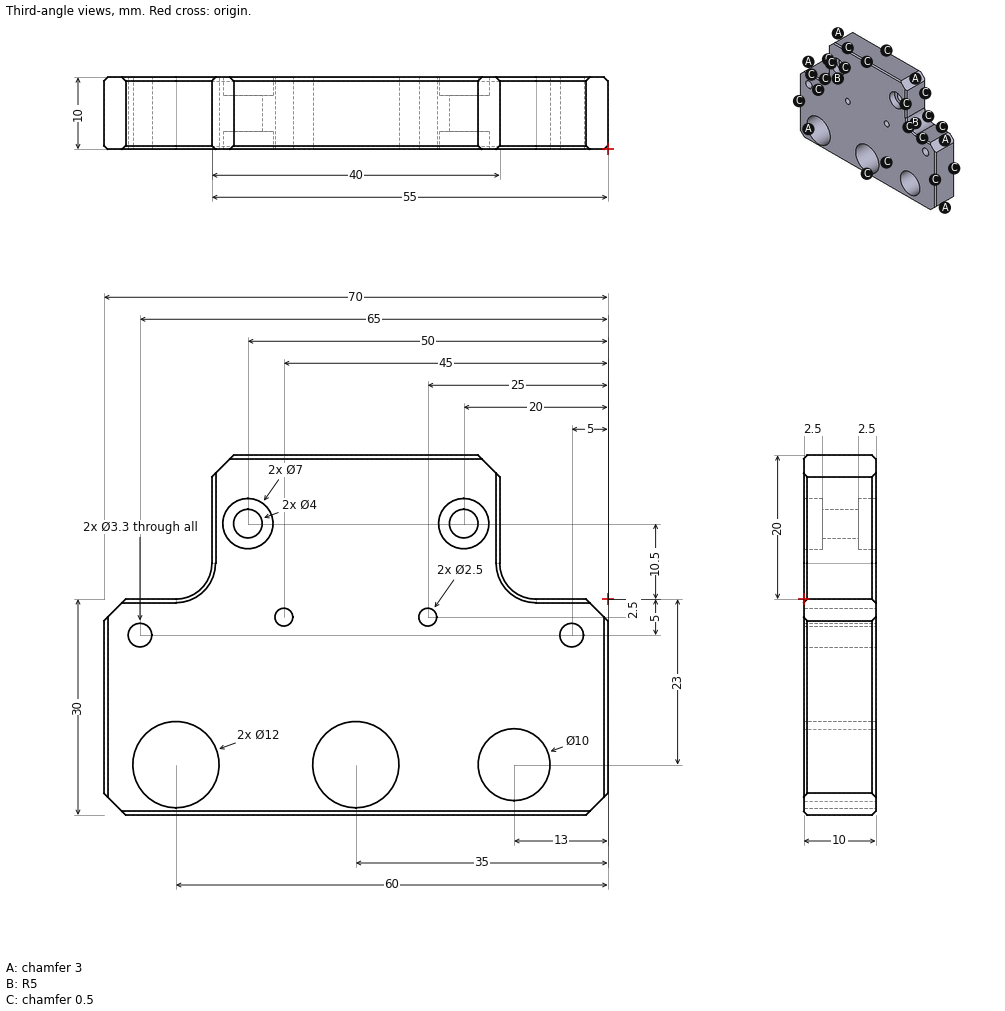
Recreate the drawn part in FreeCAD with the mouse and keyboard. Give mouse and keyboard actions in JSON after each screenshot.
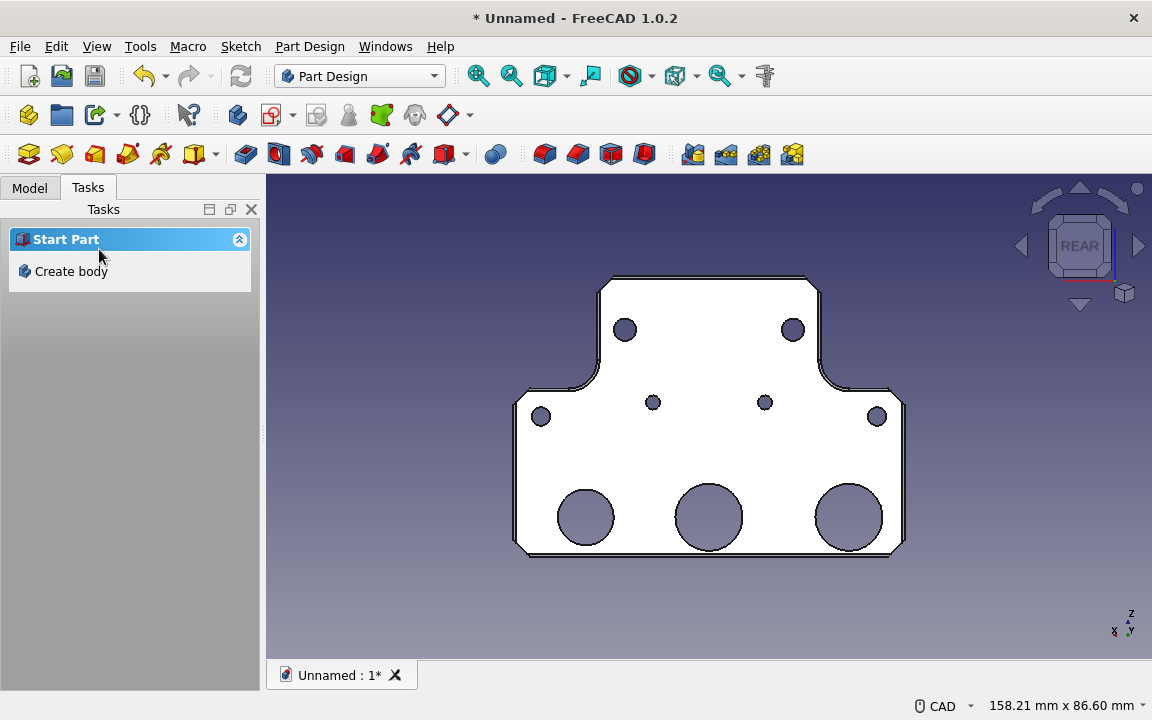
{"action": "left_click", "coordinate": [709, 337]}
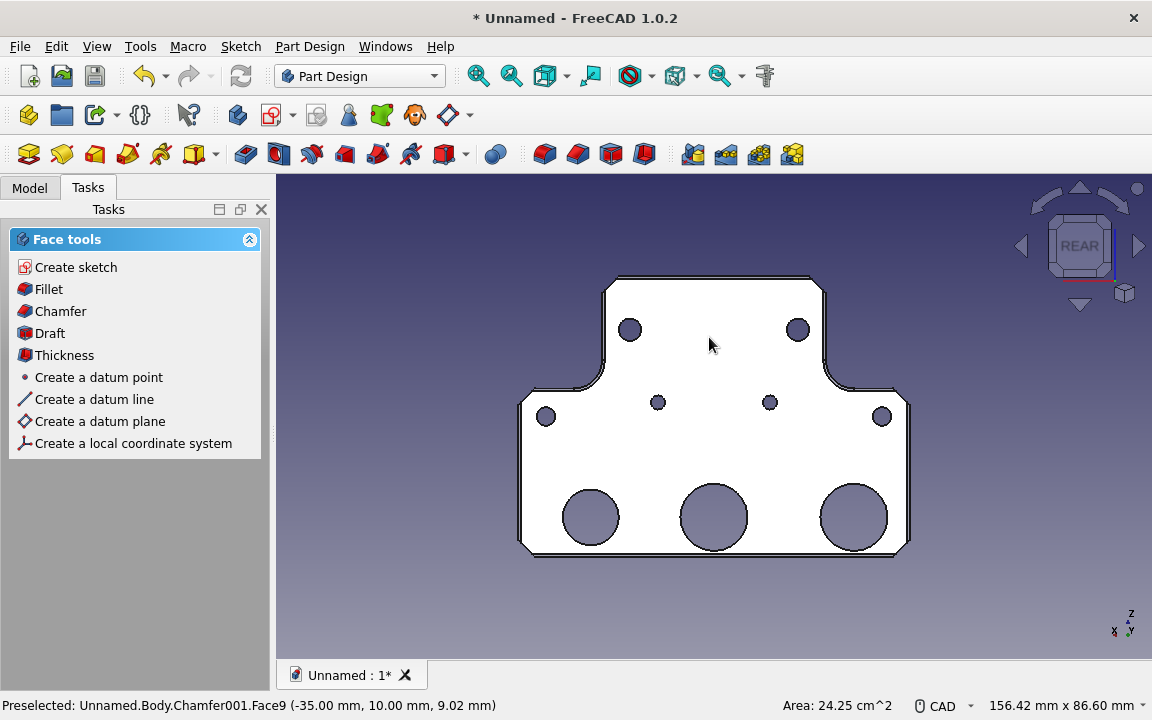
{"action": "left_click", "coordinate": [270, 116]}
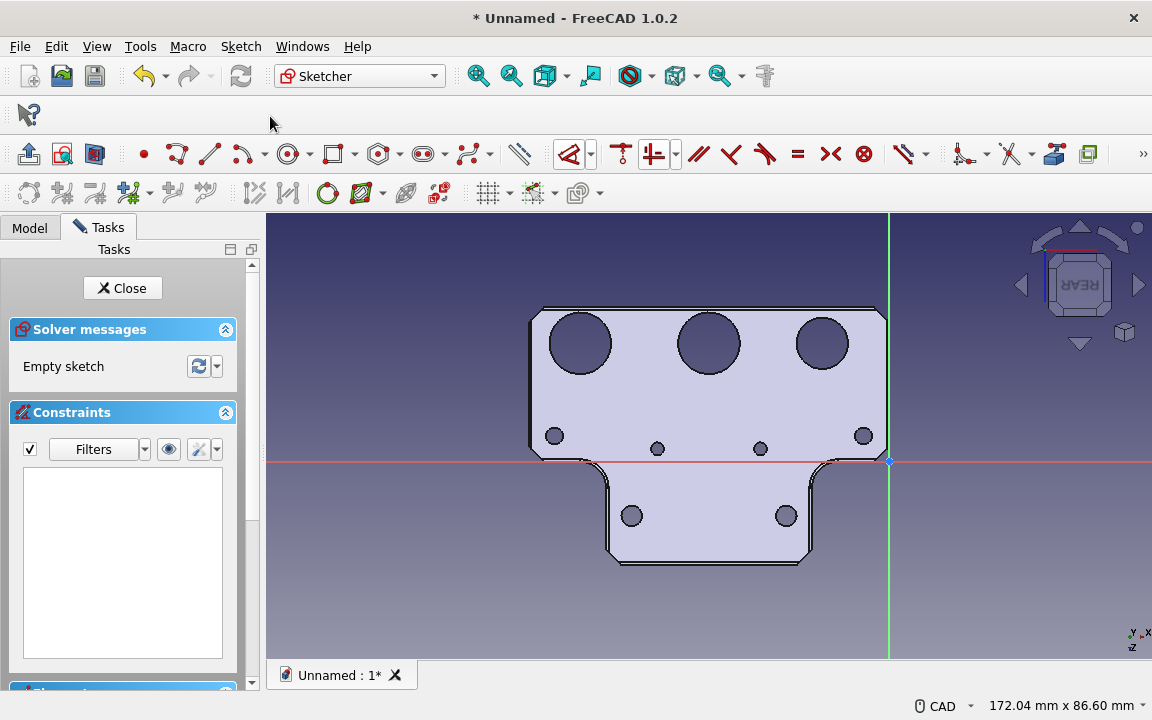
{"action": "scroll", "coordinate": [886, 573], "scroll_direction": "up", "scroll_amount": 3}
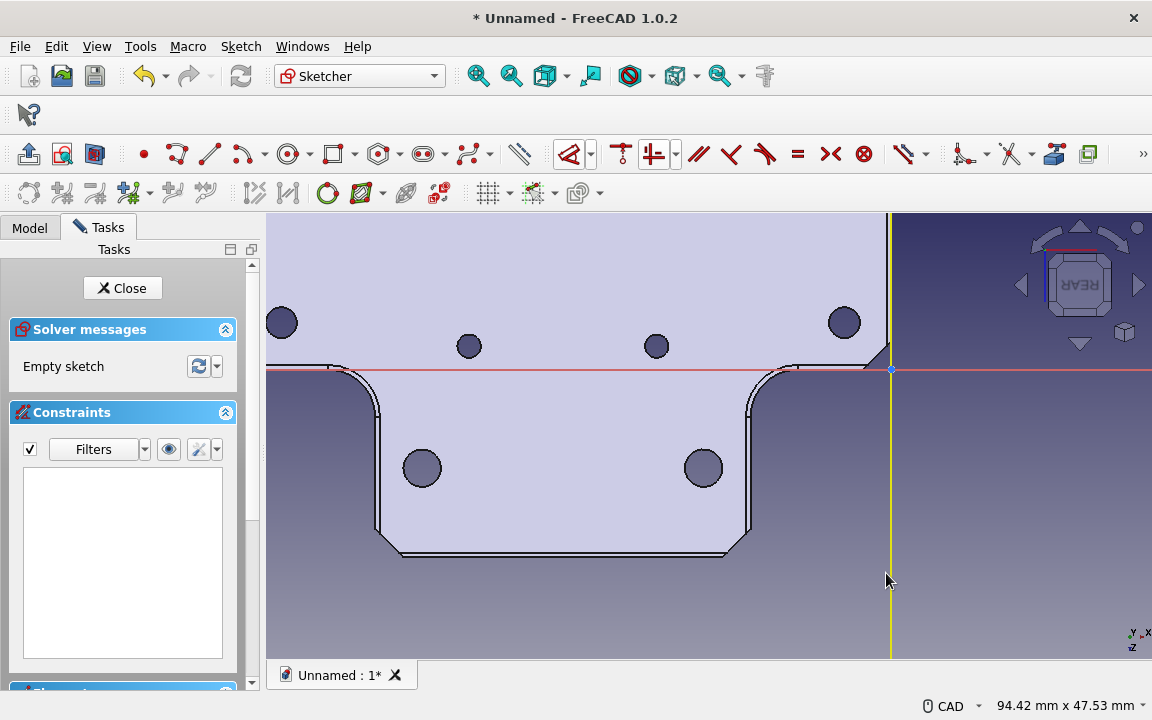
{"action": "left_click", "coordinate": [288, 154]}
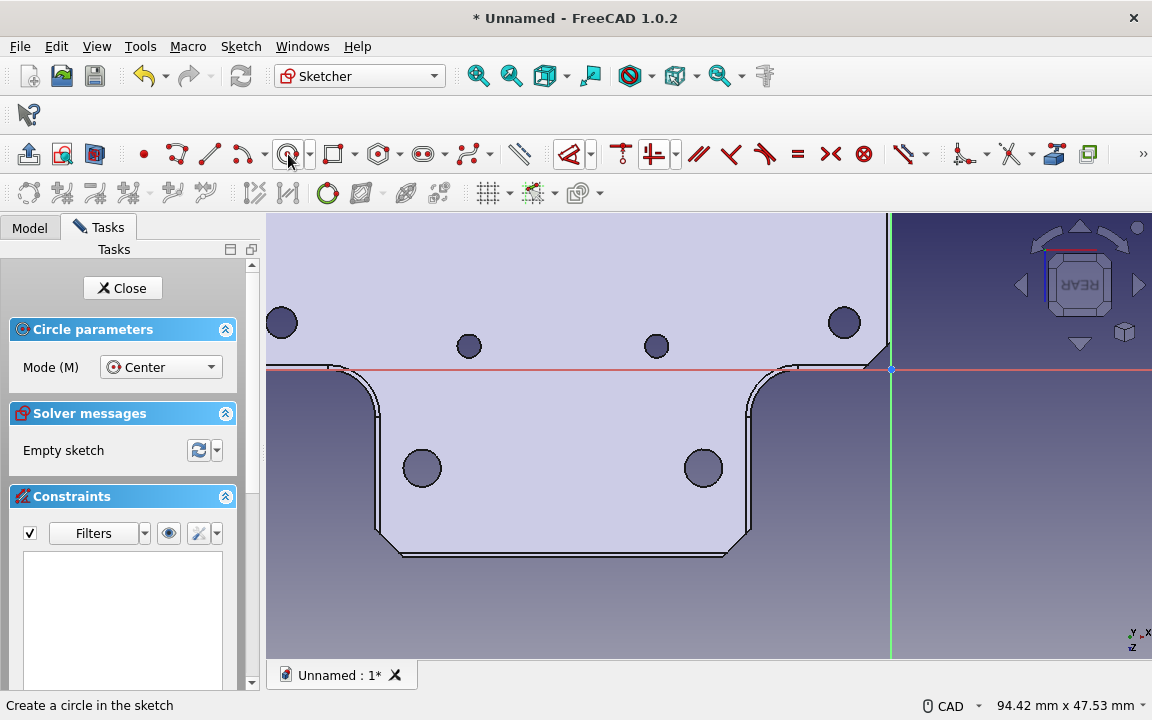
{"action": "left_click", "coordinate": [422, 468]}
{"action": "left_click", "coordinate": [445, 445]}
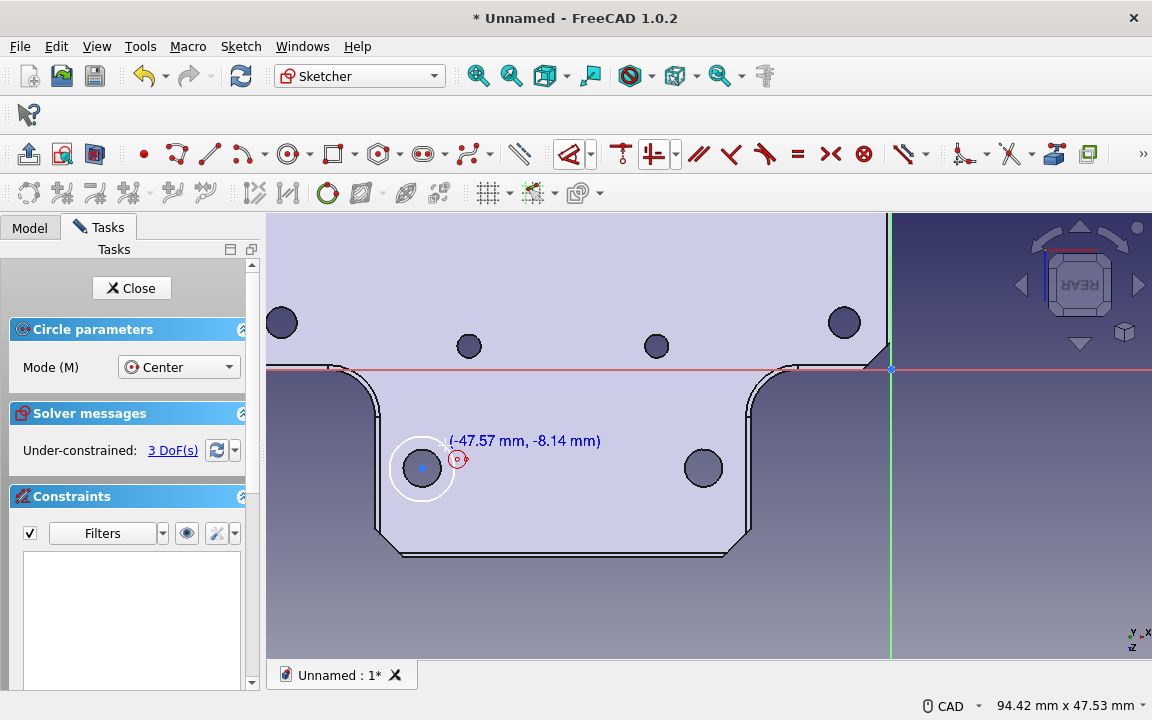
{"action": "left_click", "coordinate": [704, 468]}
{"action": "left_click", "coordinate": [727, 445]}
{"action": "key", "text": "Escape"}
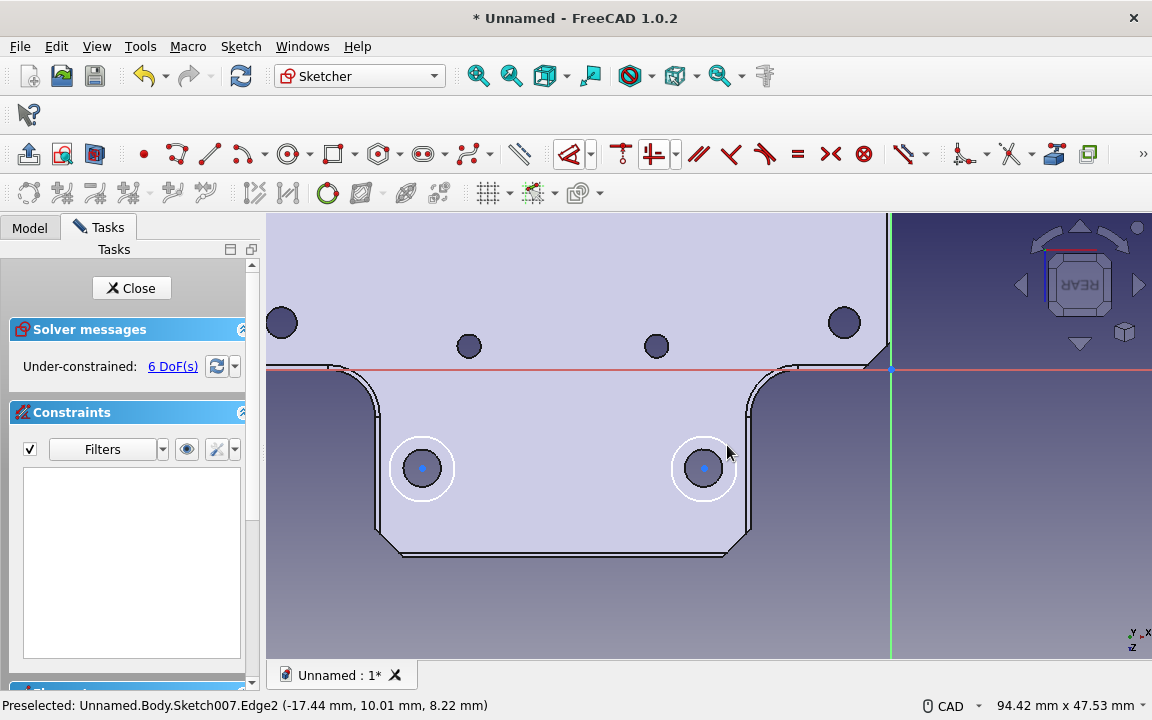
{"action": "left_click", "coordinate": [445, 446]}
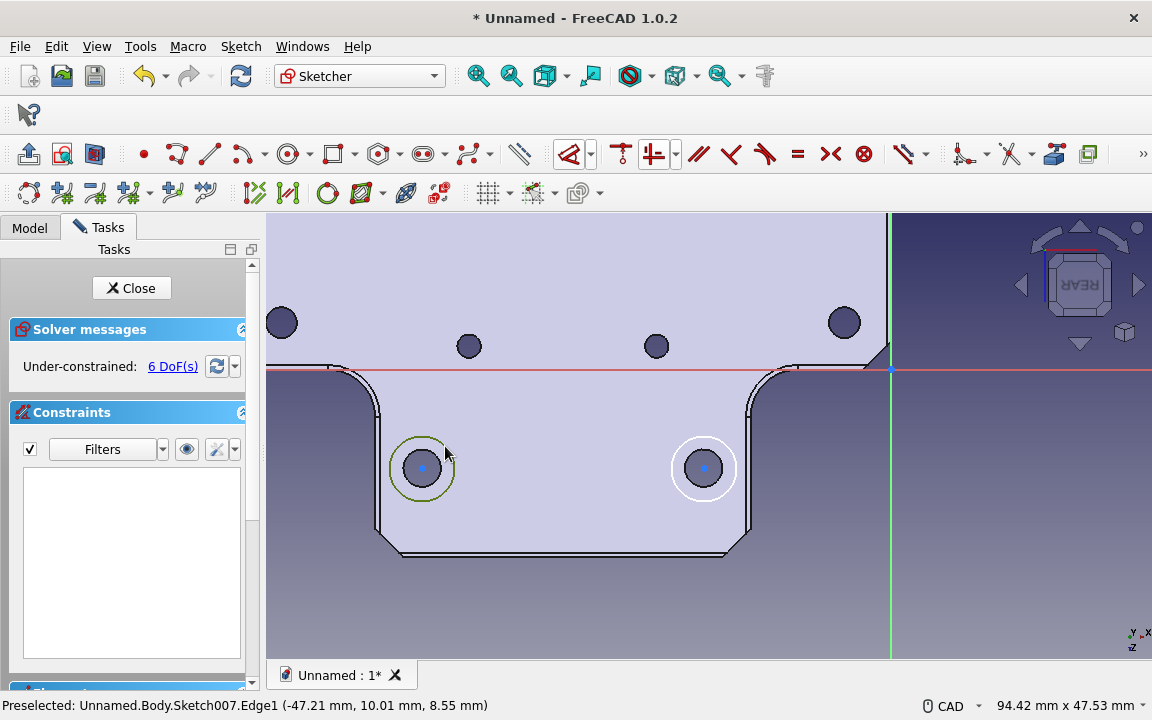
{"action": "left_click", "coordinate": [727, 446]}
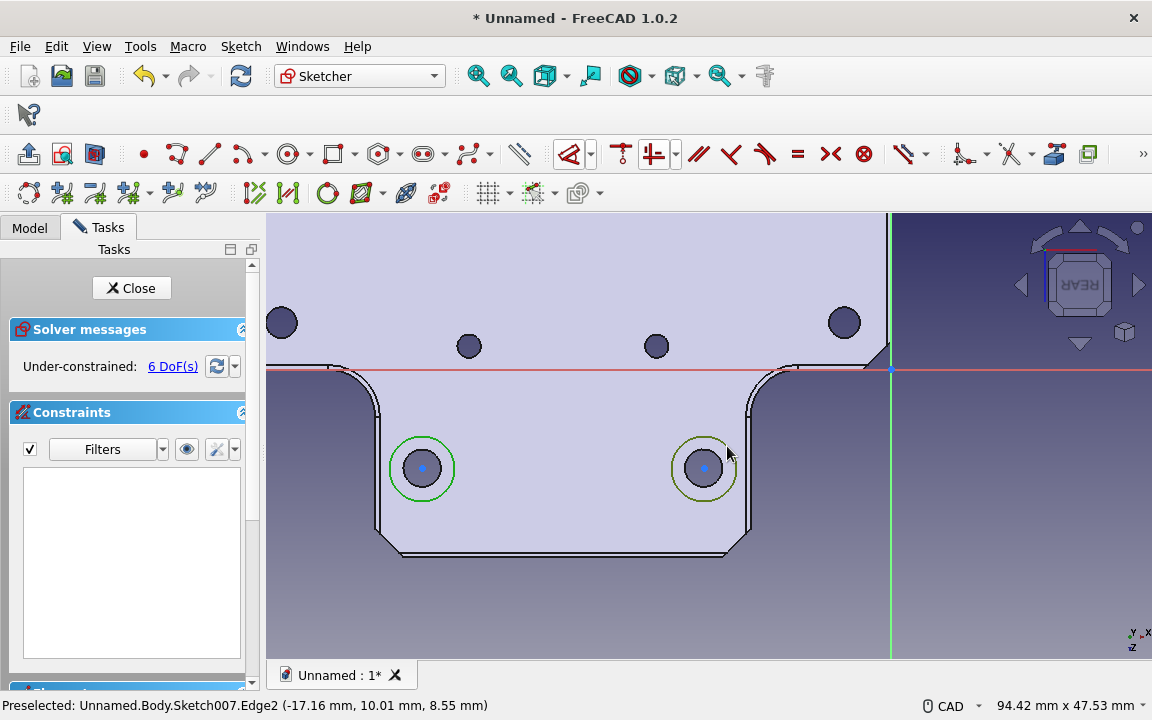
{"action": "left_click", "coordinate": [798, 154]}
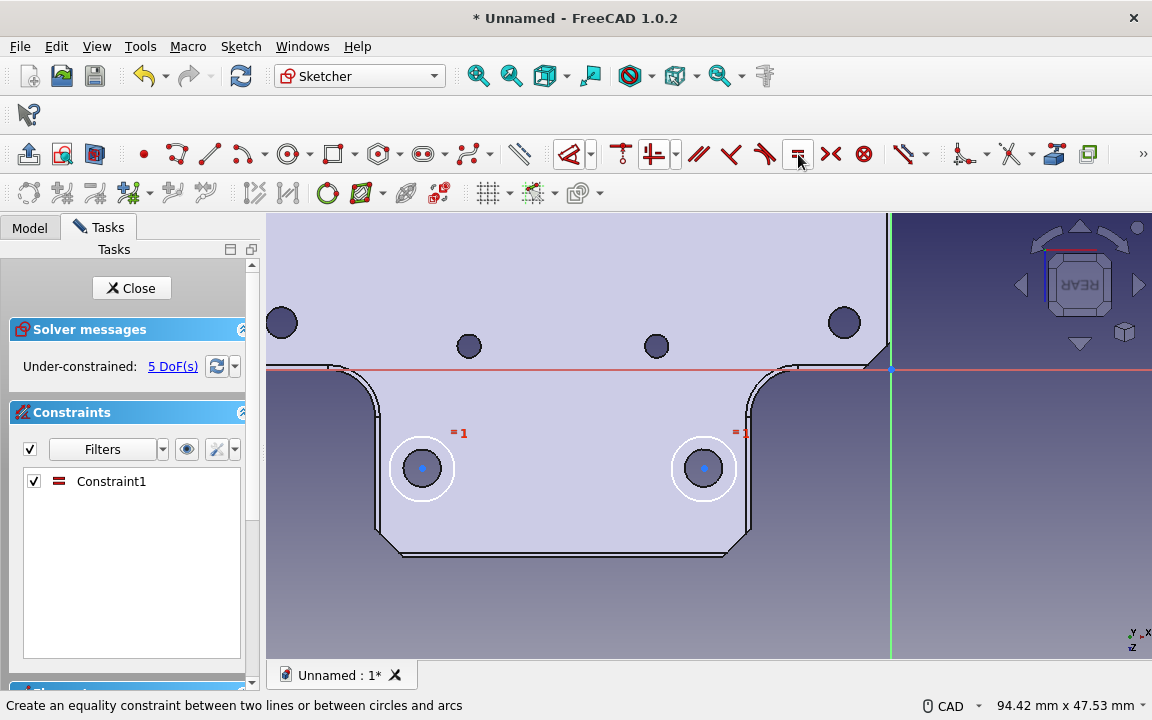
{"action": "left_click", "coordinate": [422, 469]}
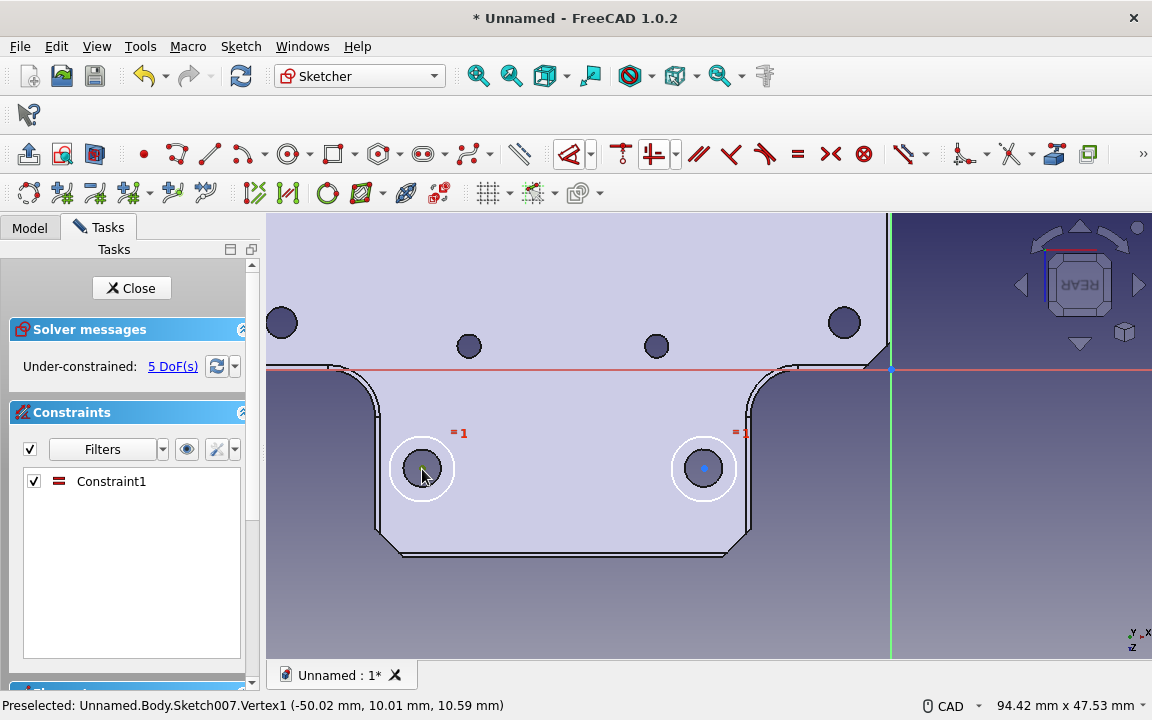
{"action": "left_click", "coordinate": [704, 469]}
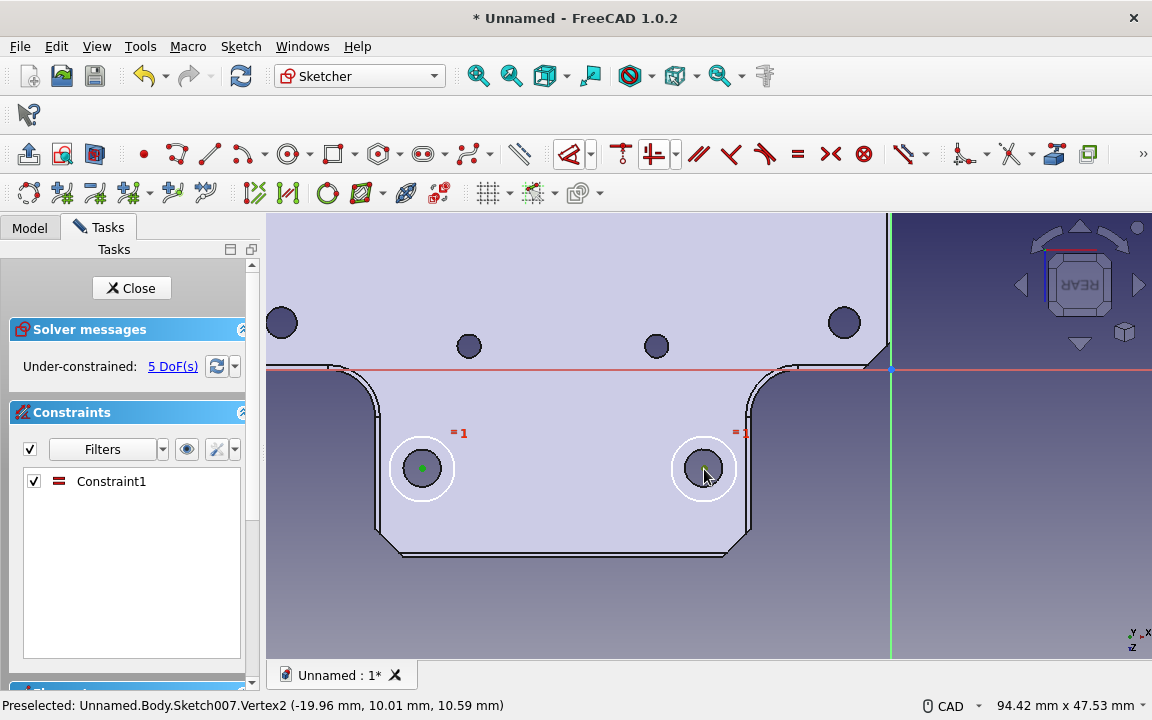
{"action": "left_click", "coordinate": [676, 154]}